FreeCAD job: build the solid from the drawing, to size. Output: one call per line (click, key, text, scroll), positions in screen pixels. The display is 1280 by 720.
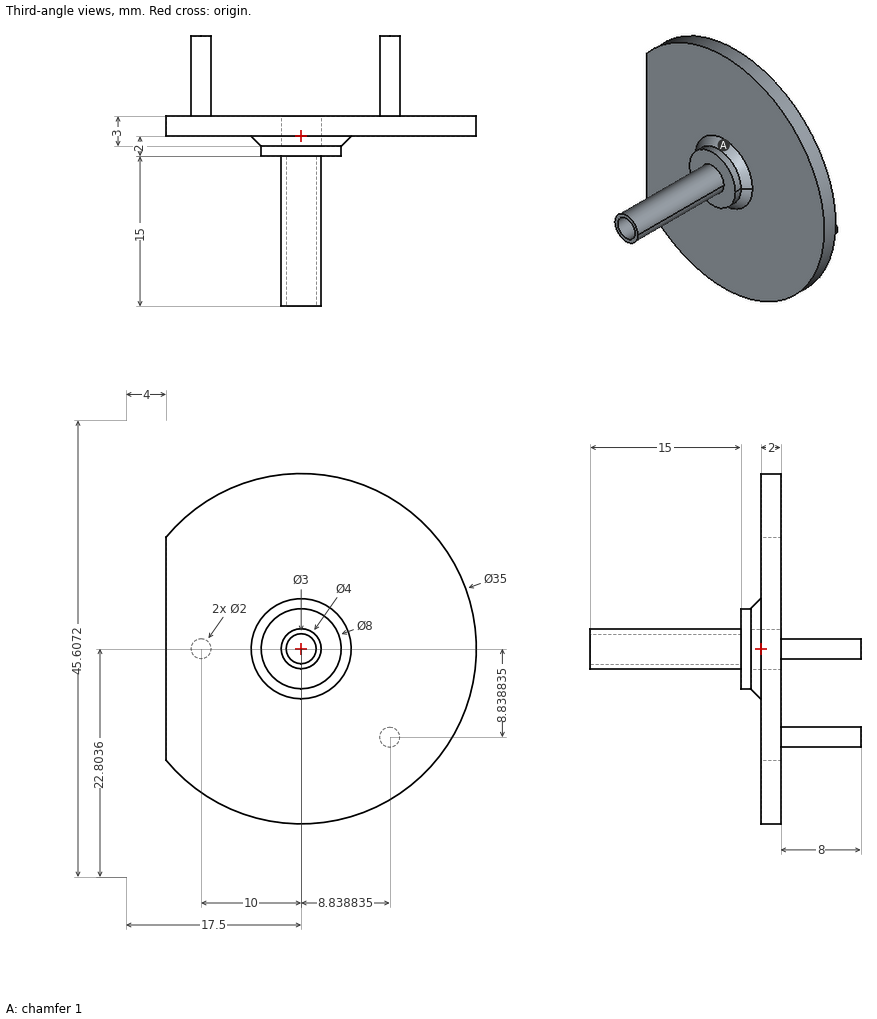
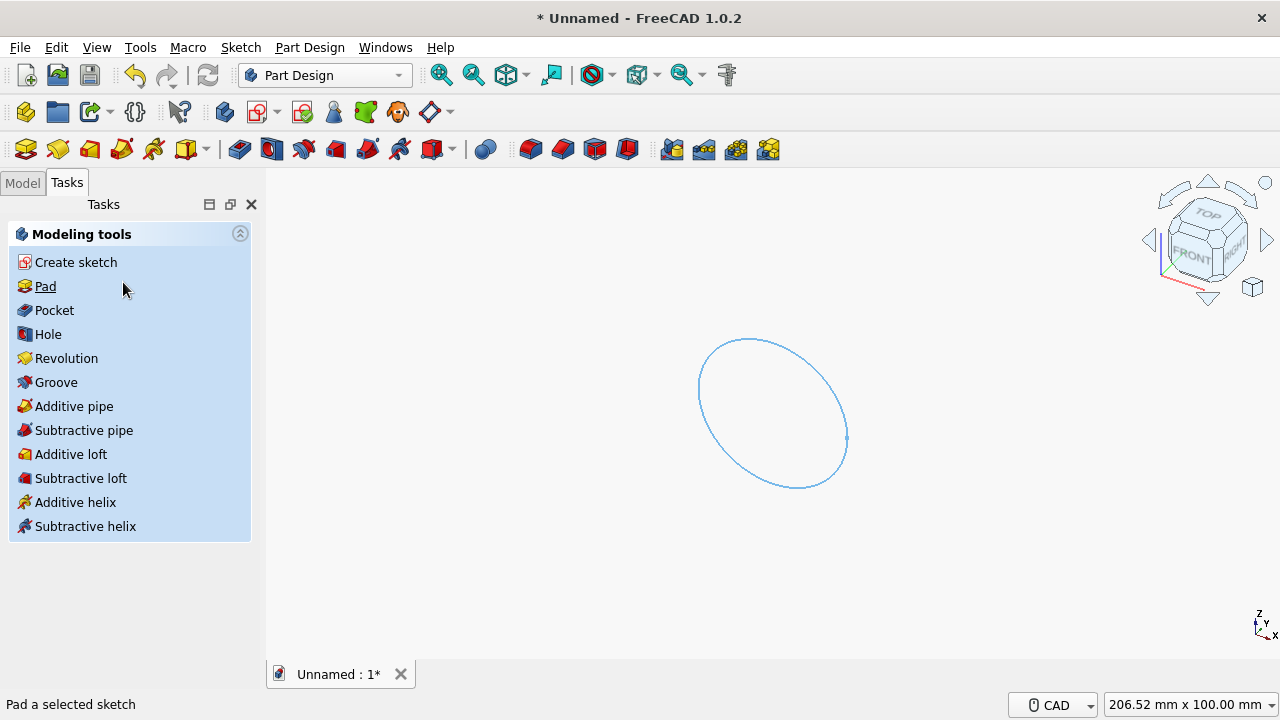
click(26, 150)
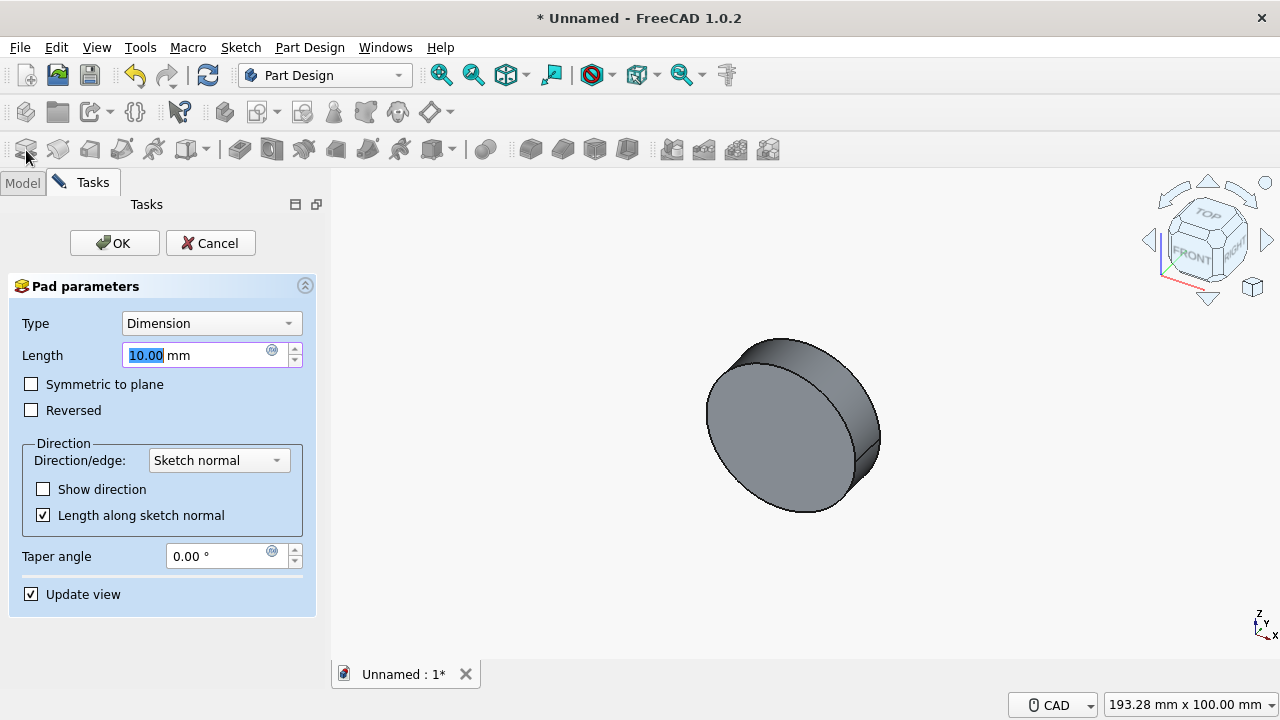
text(2)
key(Tab)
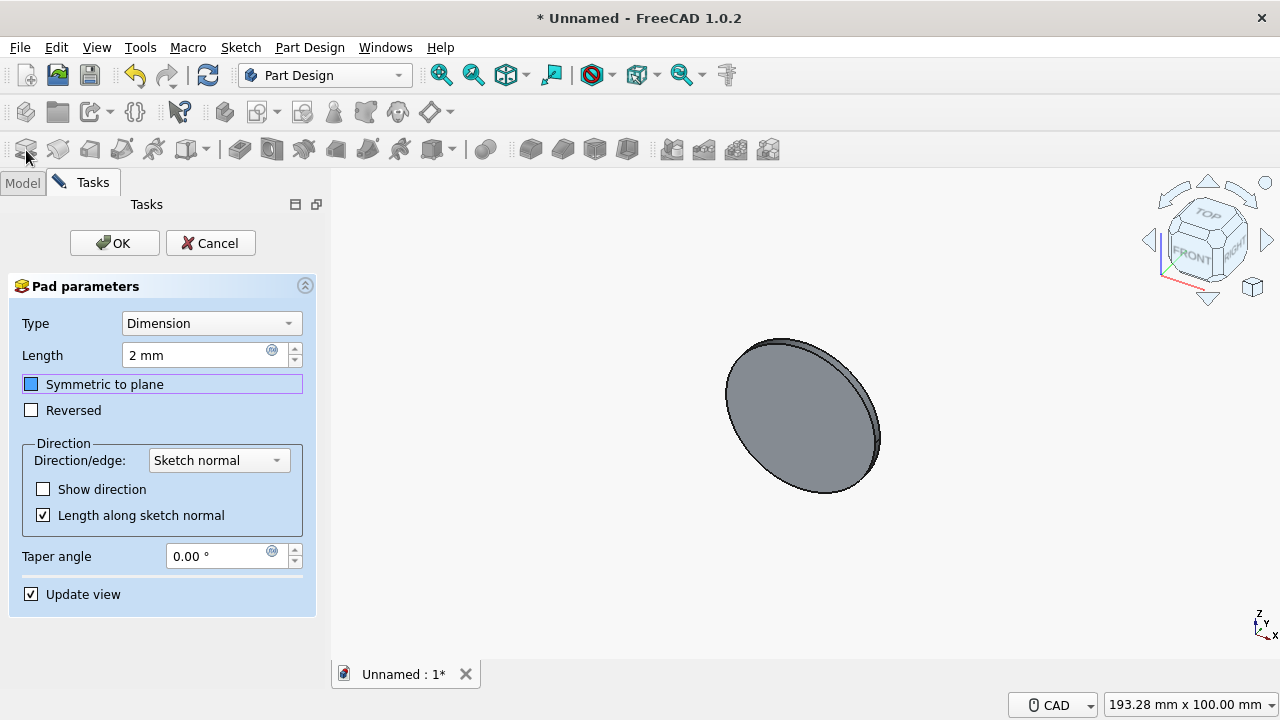
click(30, 410)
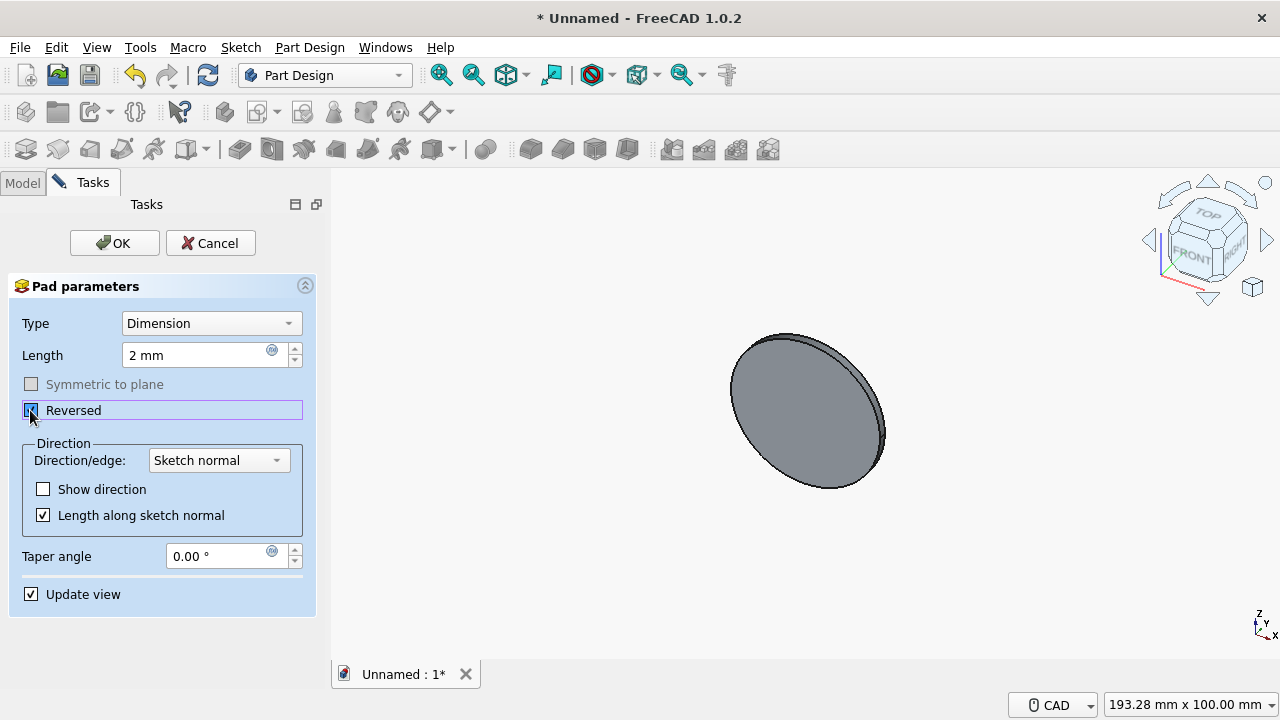
click(115, 243)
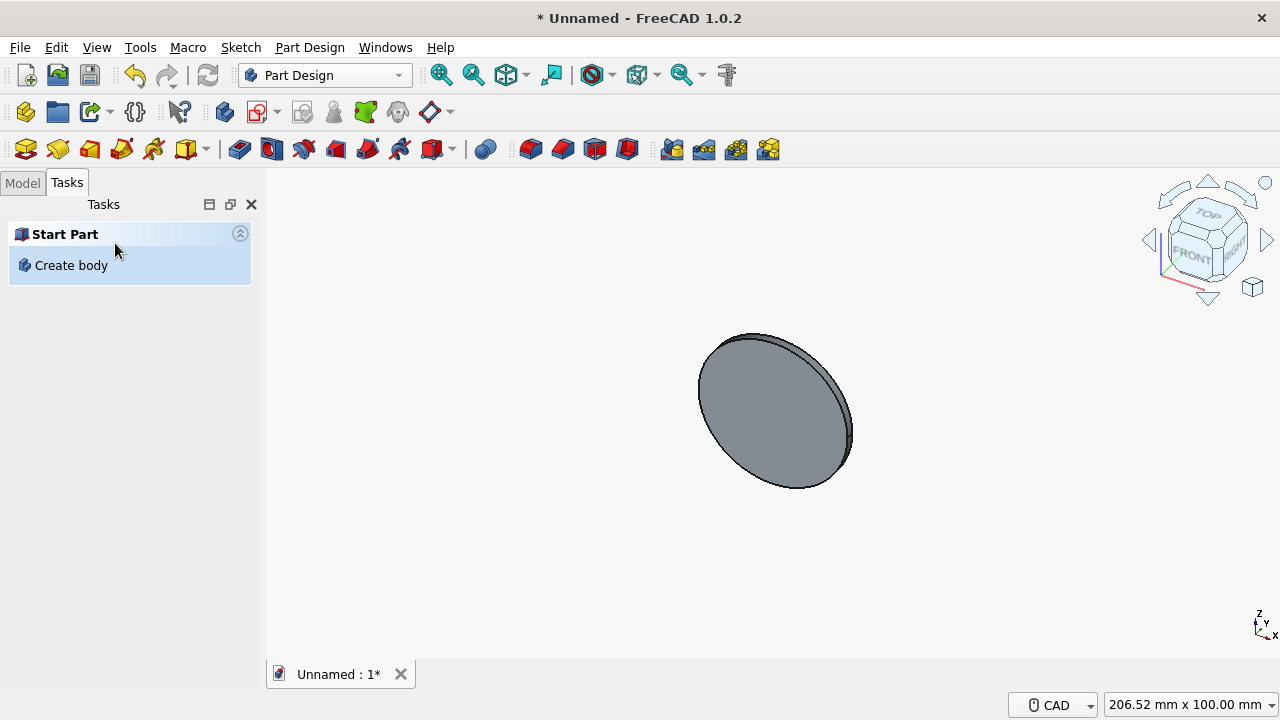
click(442, 76)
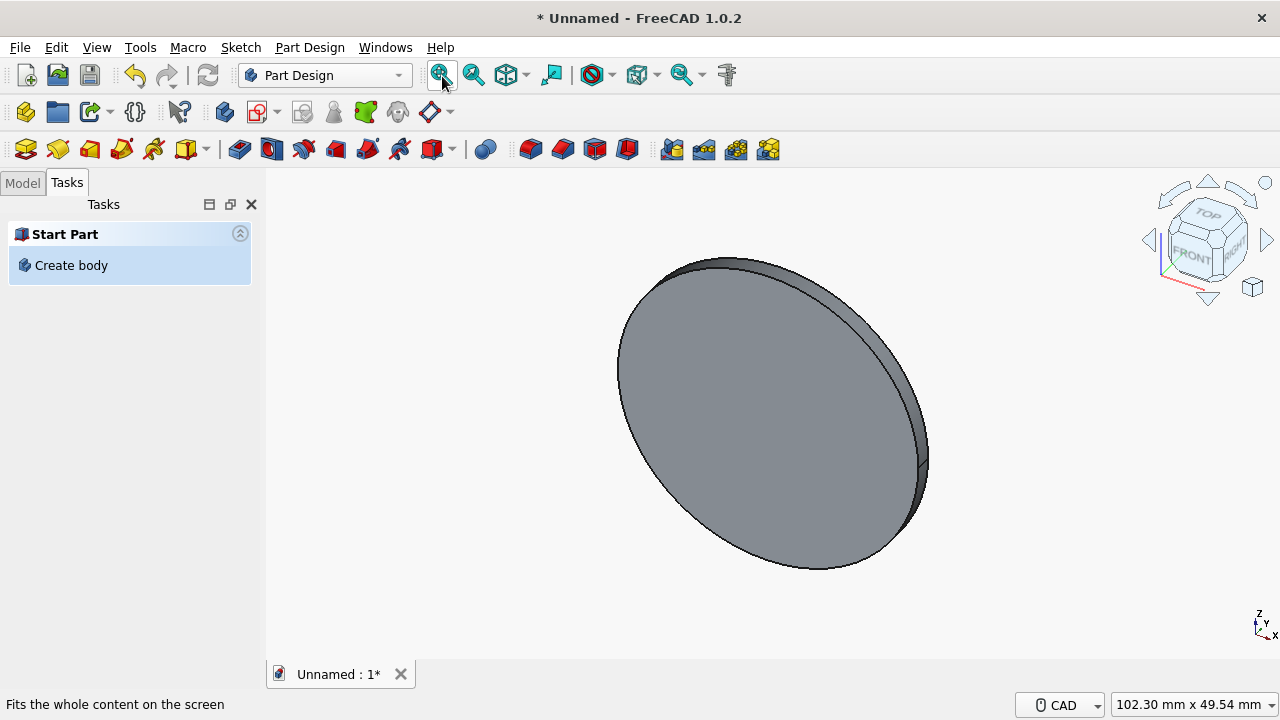
click(258, 112)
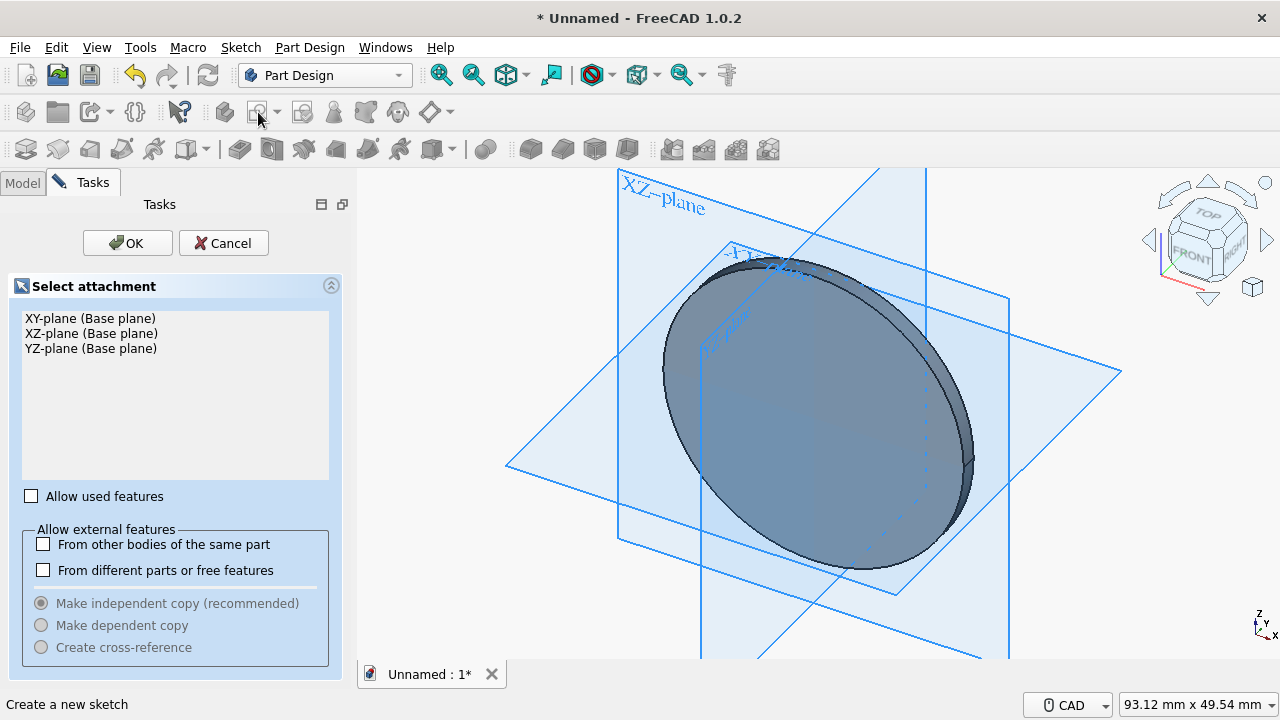
click(82, 334)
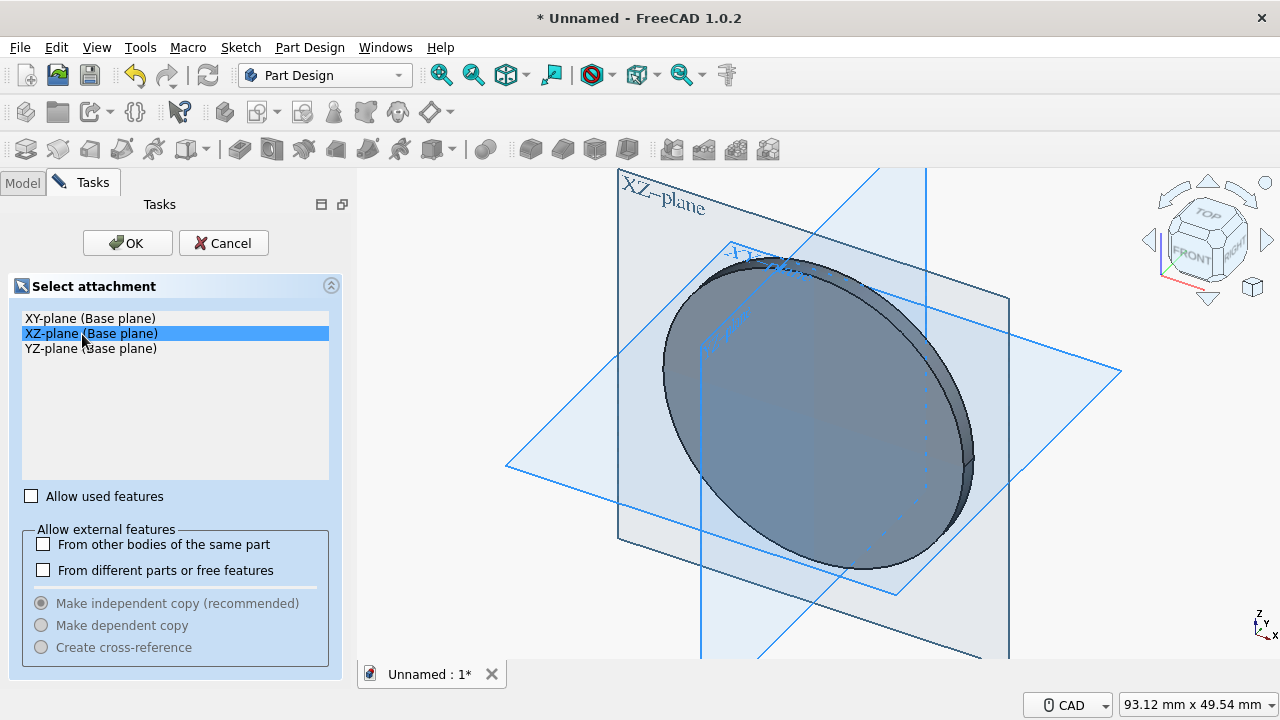
click(128, 243)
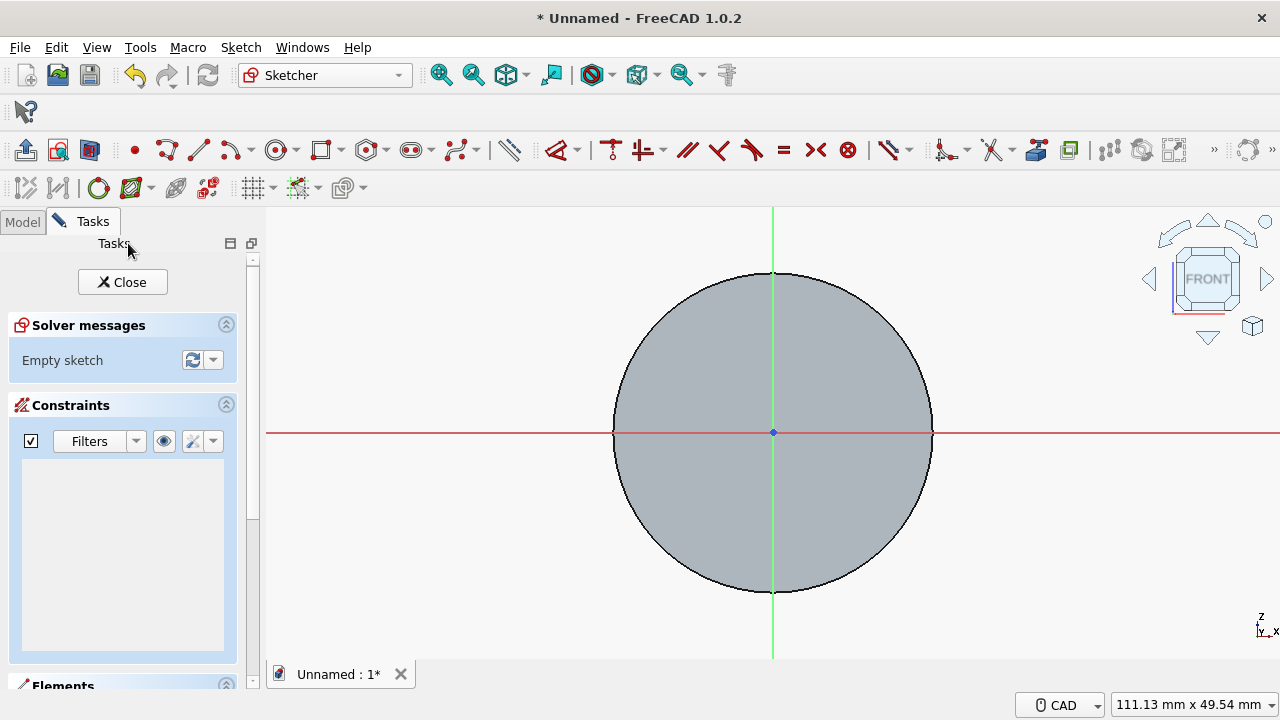
scroll(795, 433, up, 7)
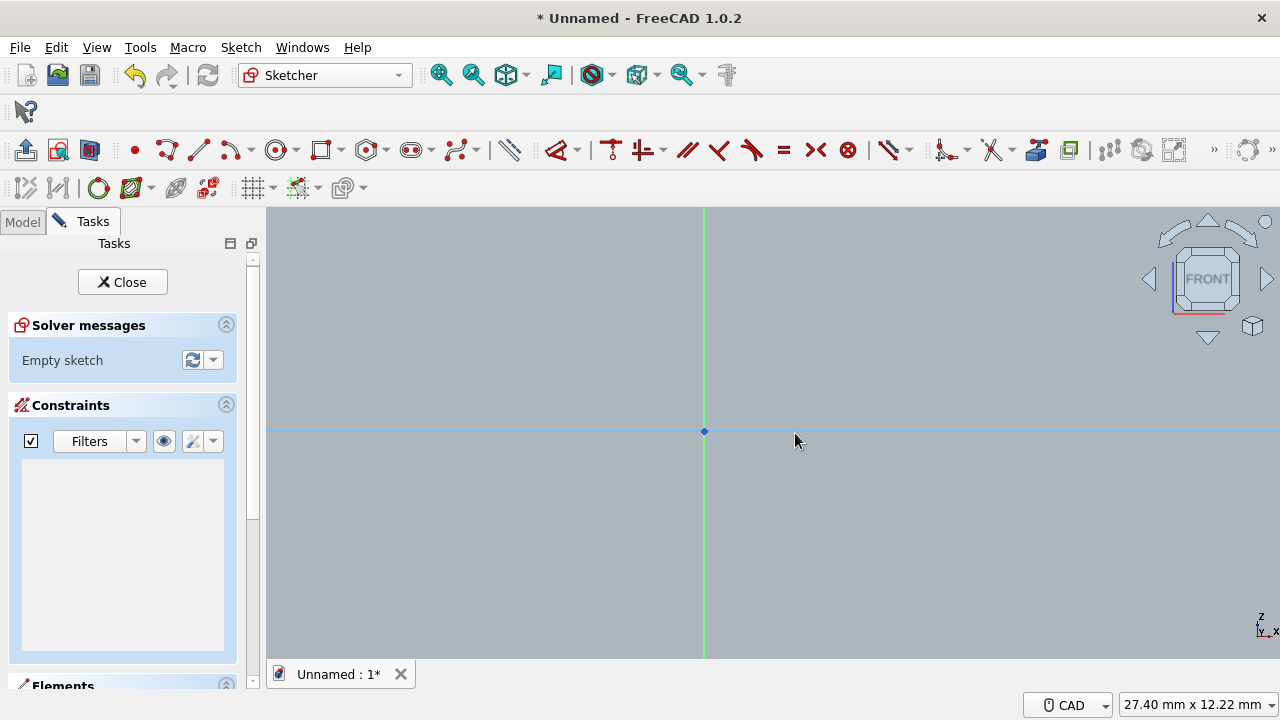
click(276, 150)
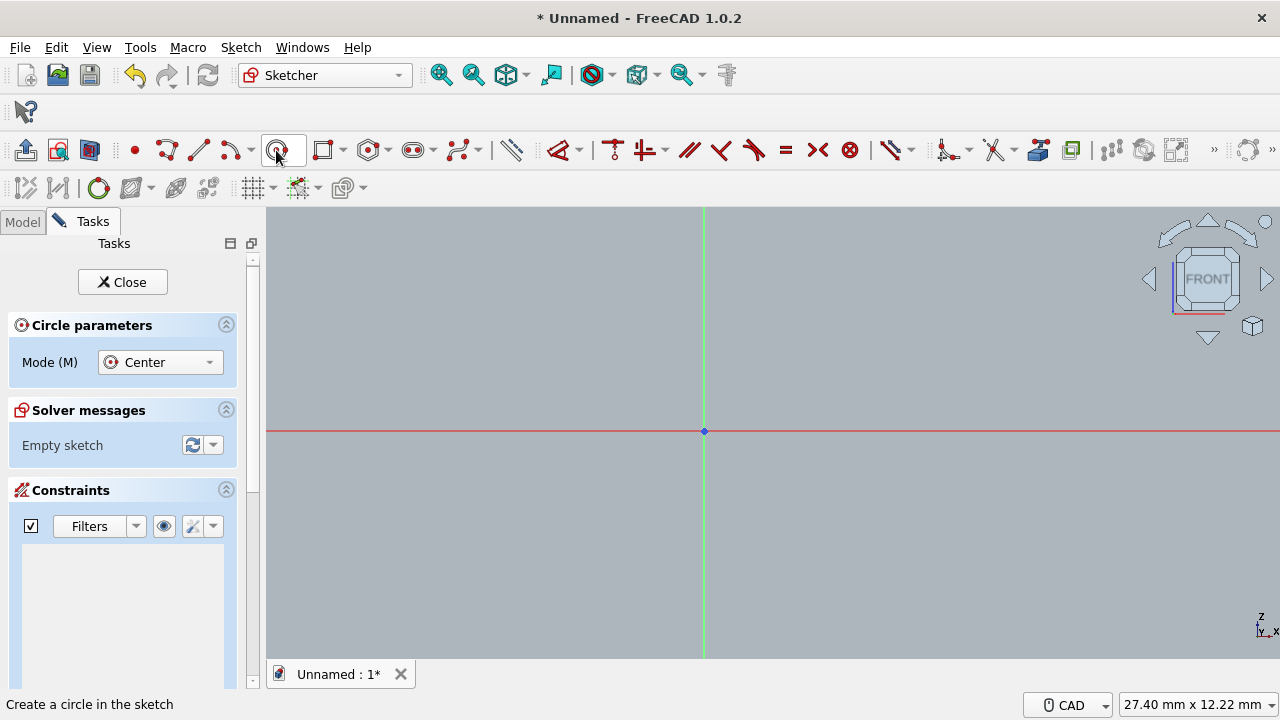
click(704, 431)
click(809, 327)
key(Escape)